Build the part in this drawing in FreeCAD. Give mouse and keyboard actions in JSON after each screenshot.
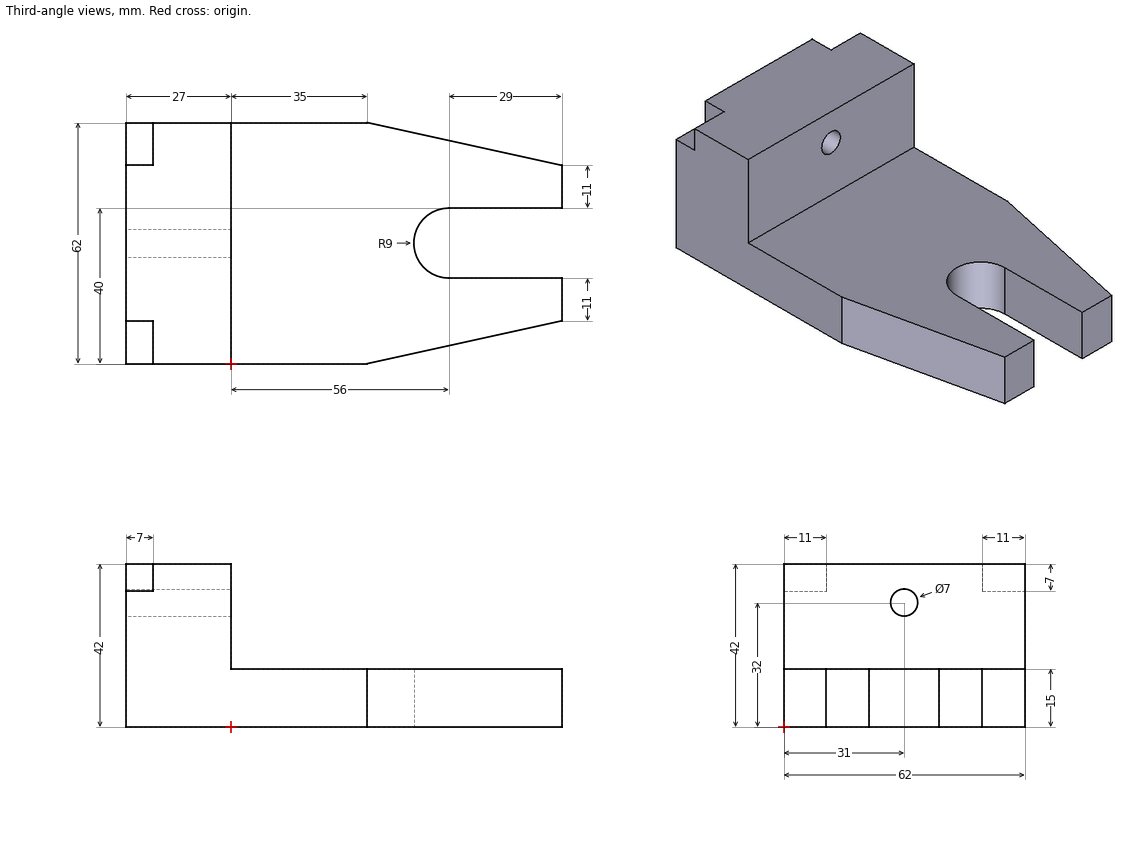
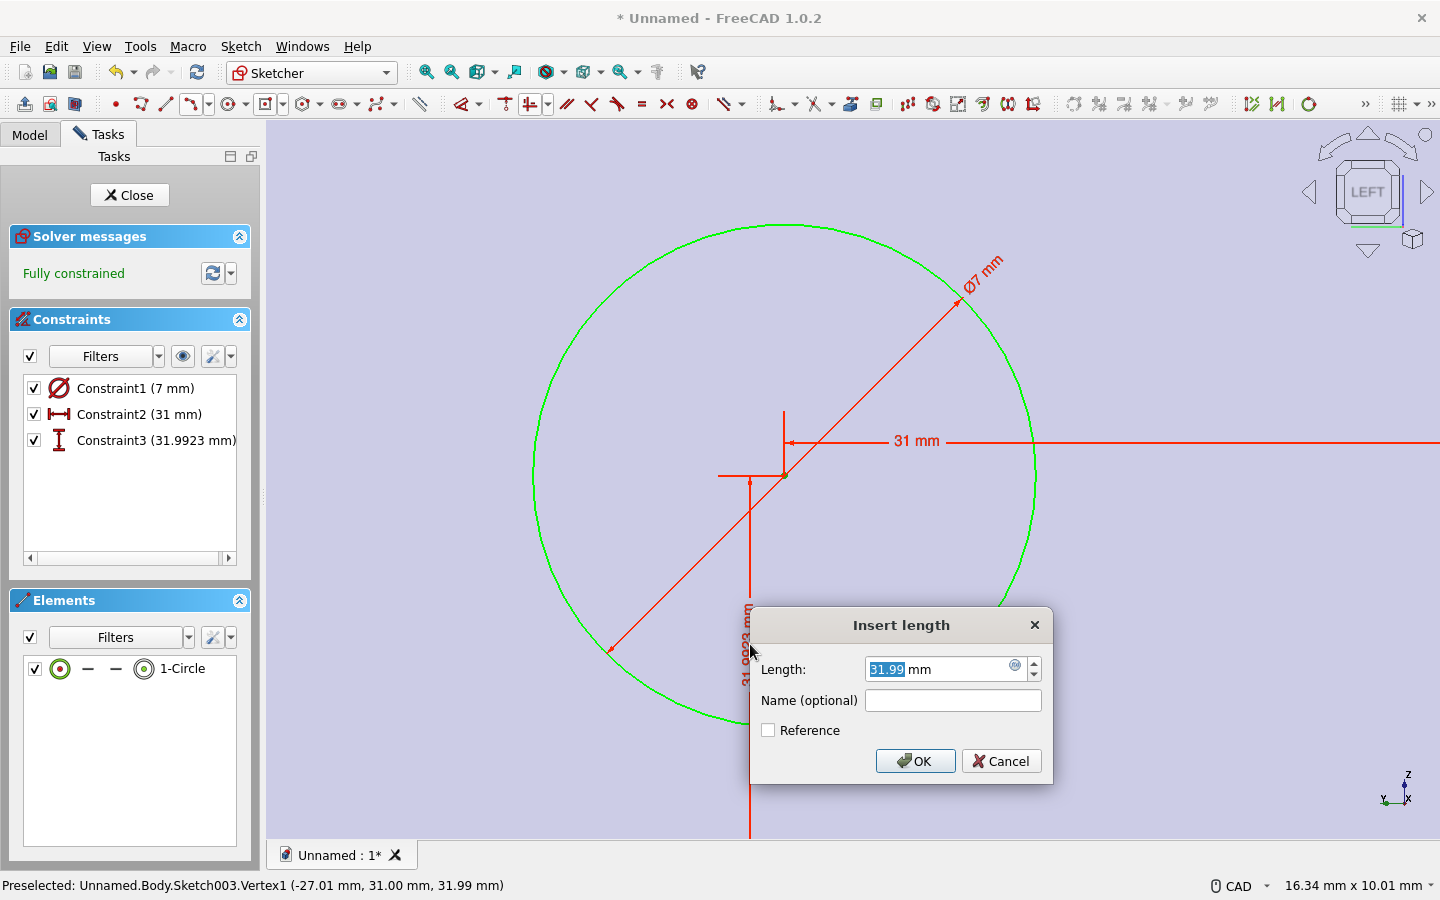
{"action": "type", "text": "32"}
{"action": "key", "text": "Return"}
{"action": "key", "text": "Escape"}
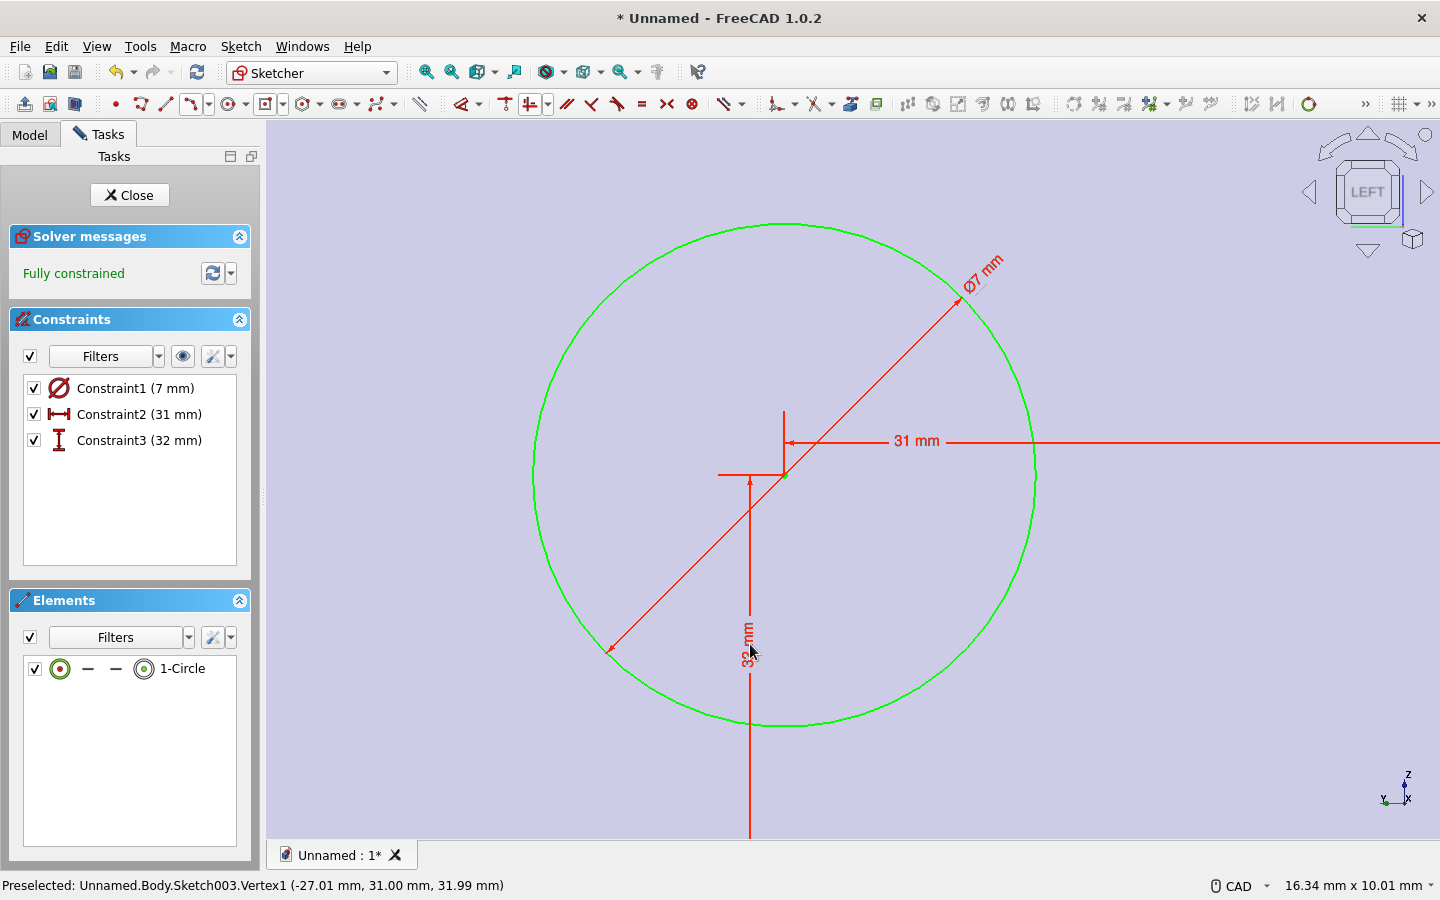
{"action": "left_click", "coordinate": [130, 195]}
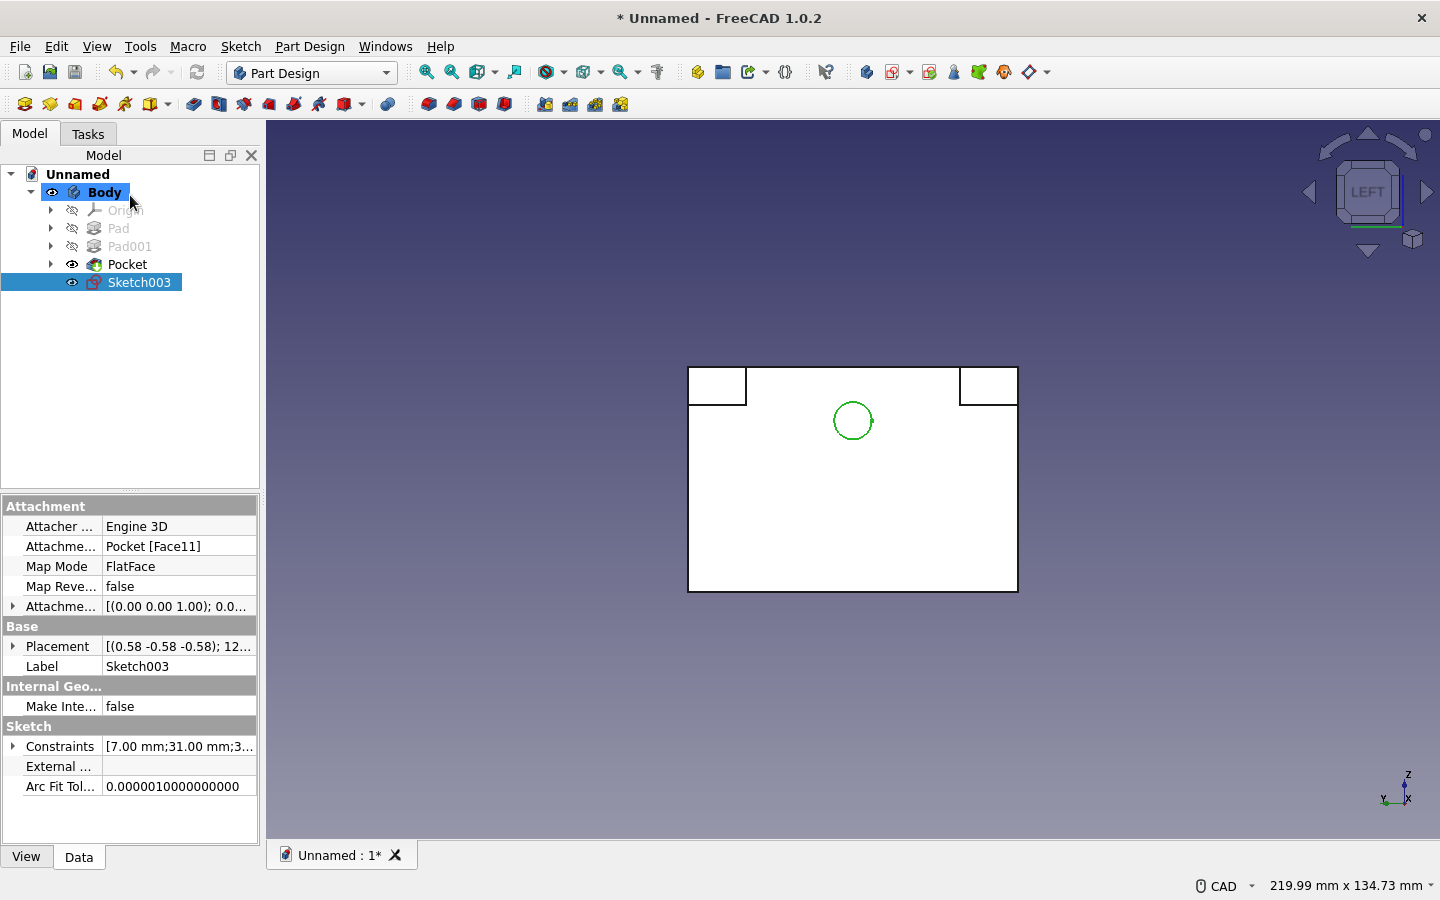
{"action": "left_click", "coordinate": [194, 104]}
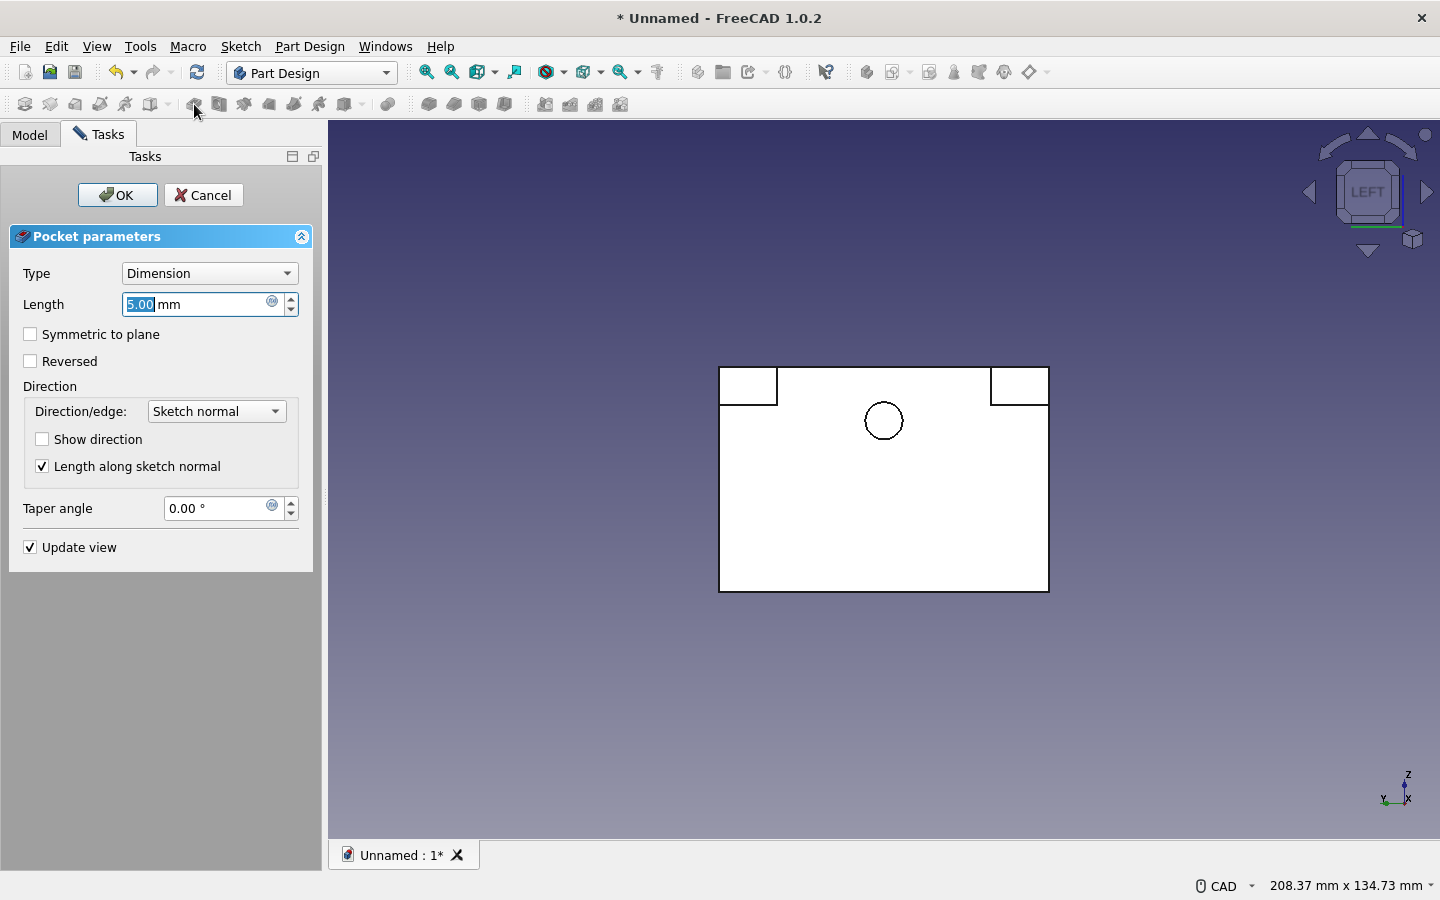
{"action": "left_click", "coordinate": [210, 274]}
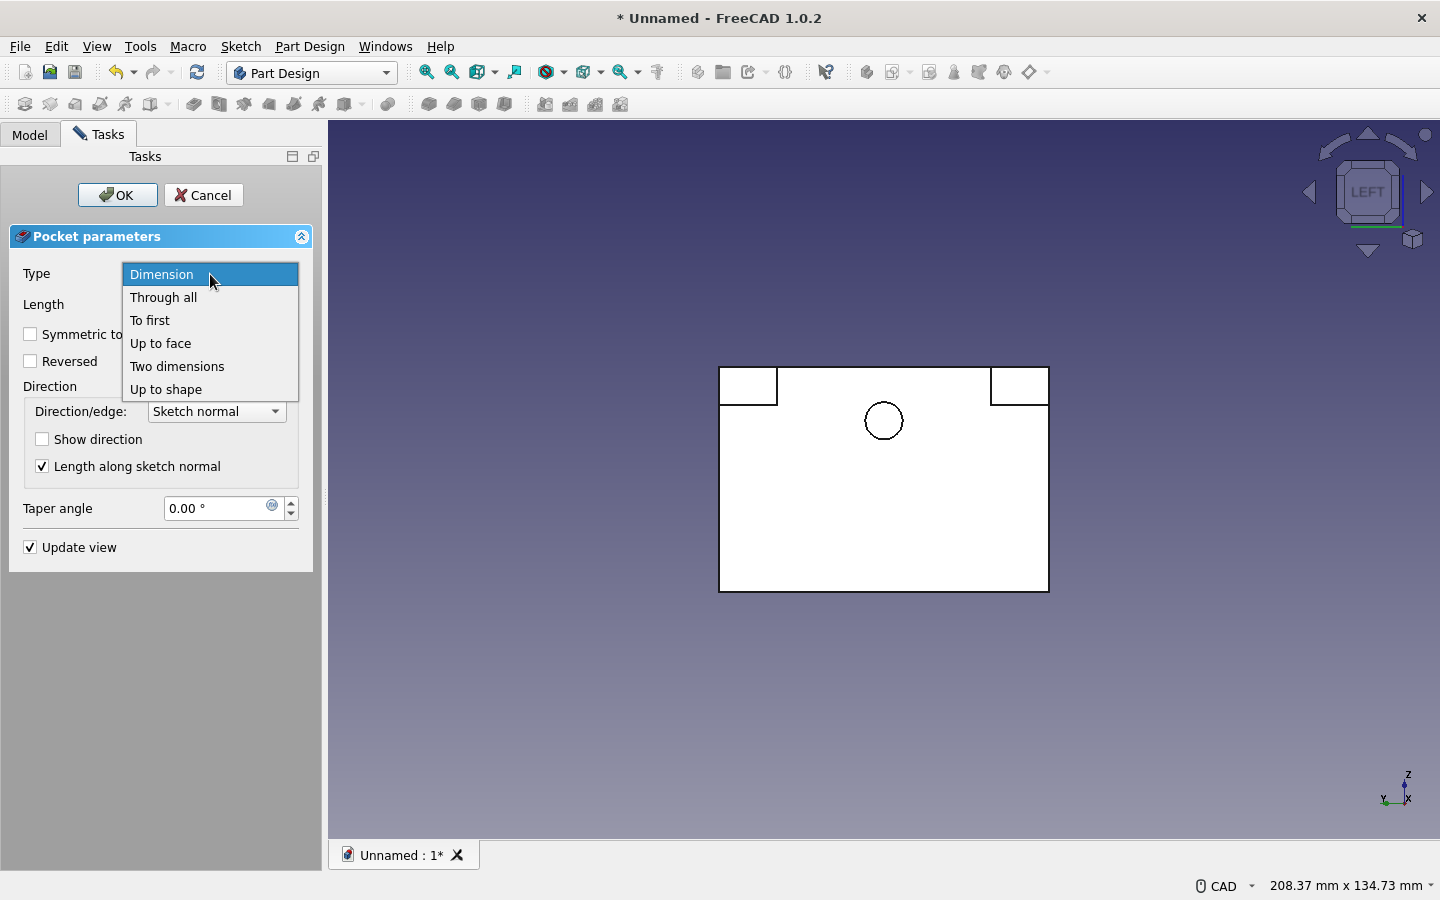
{"action": "left_click", "coordinate": [208, 298]}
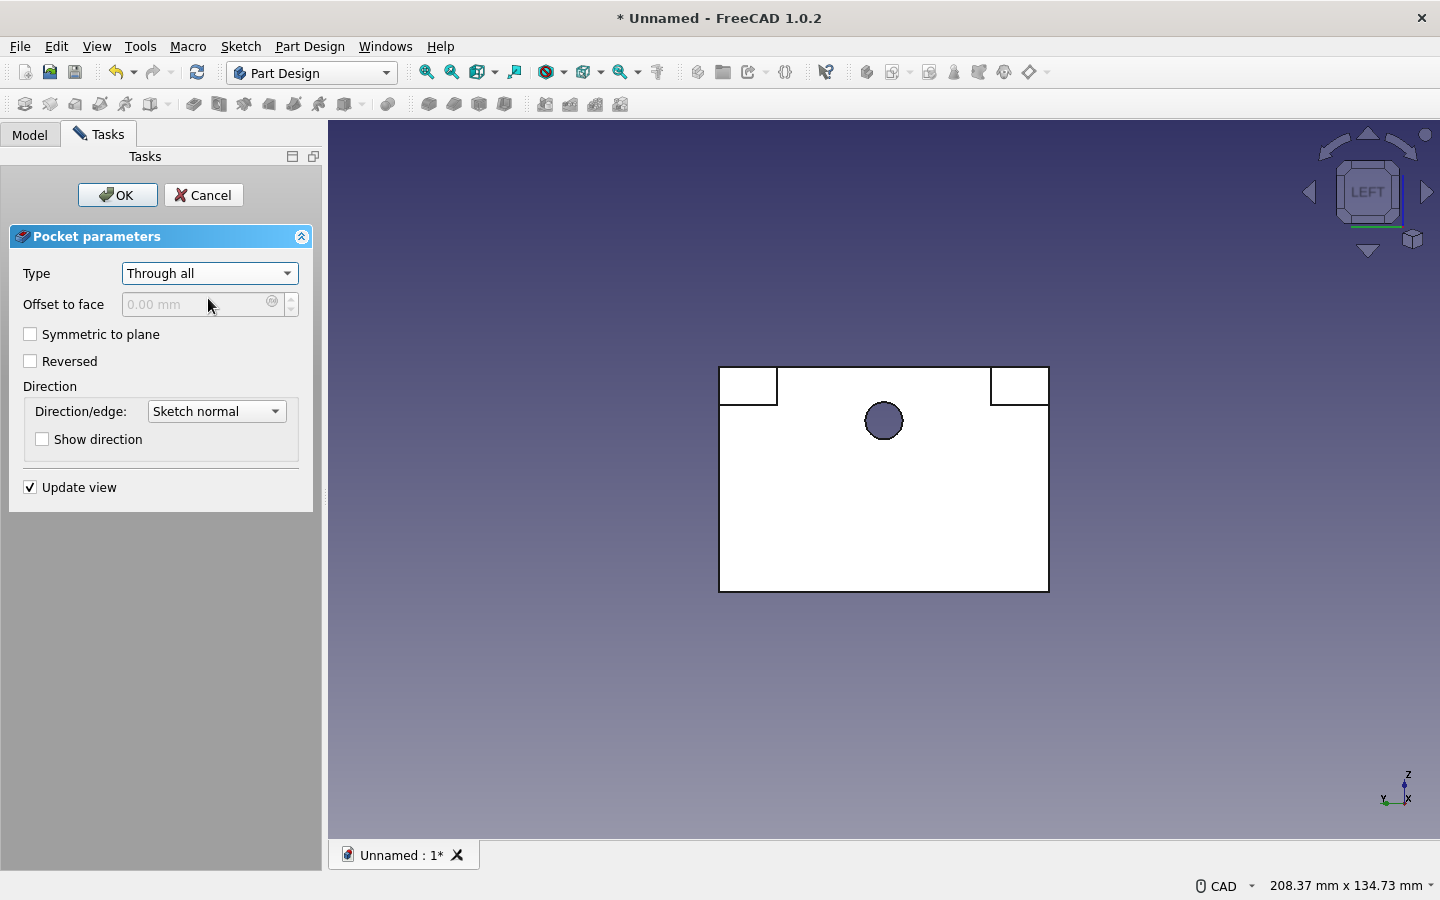
{"action": "left_click", "coordinate": [118, 195]}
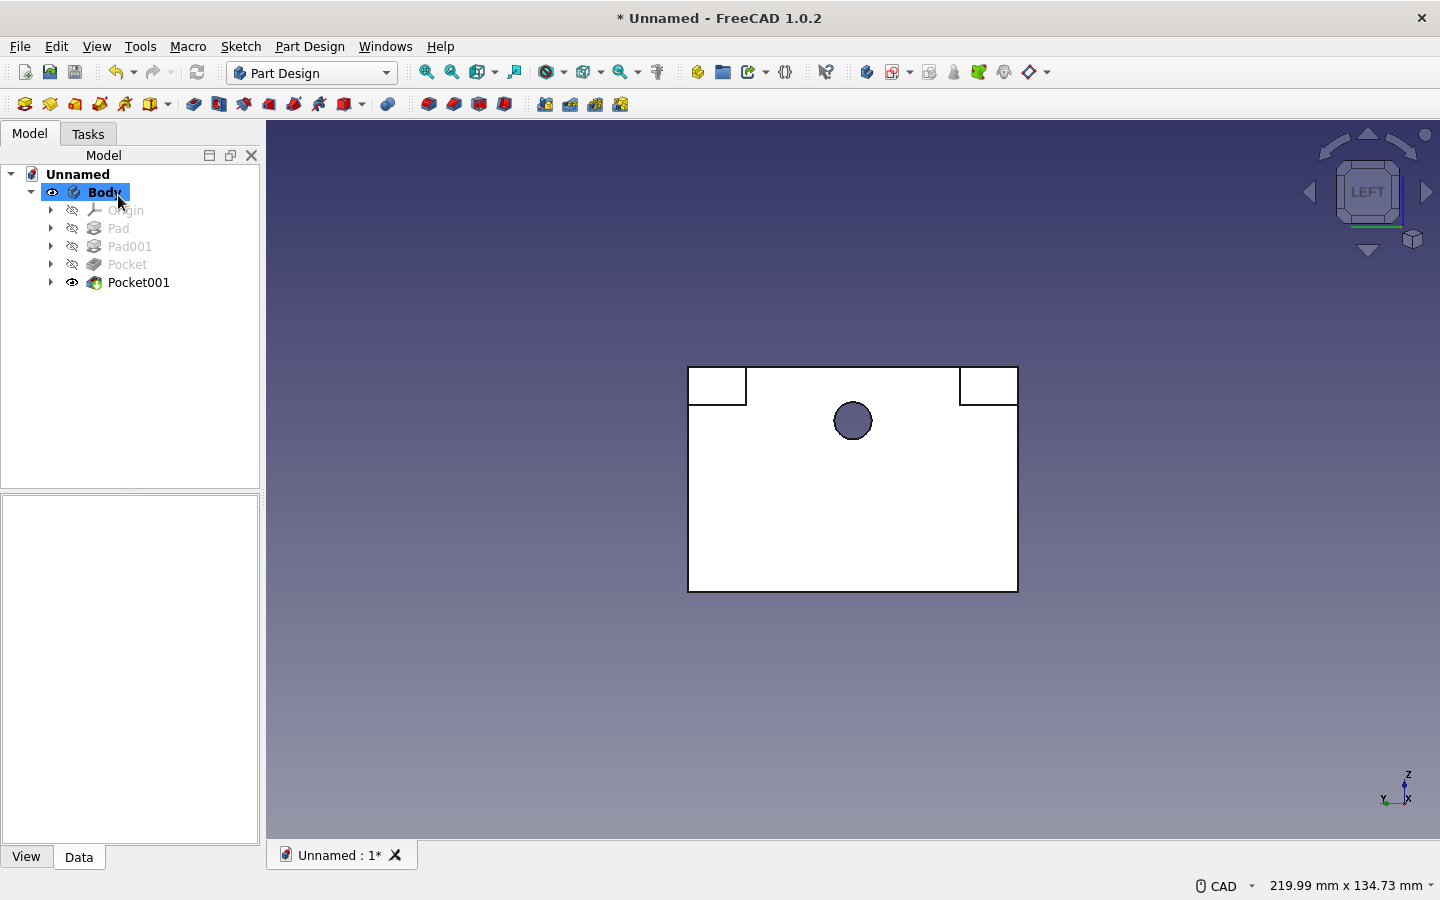
{"action": "key", "text": "0"}